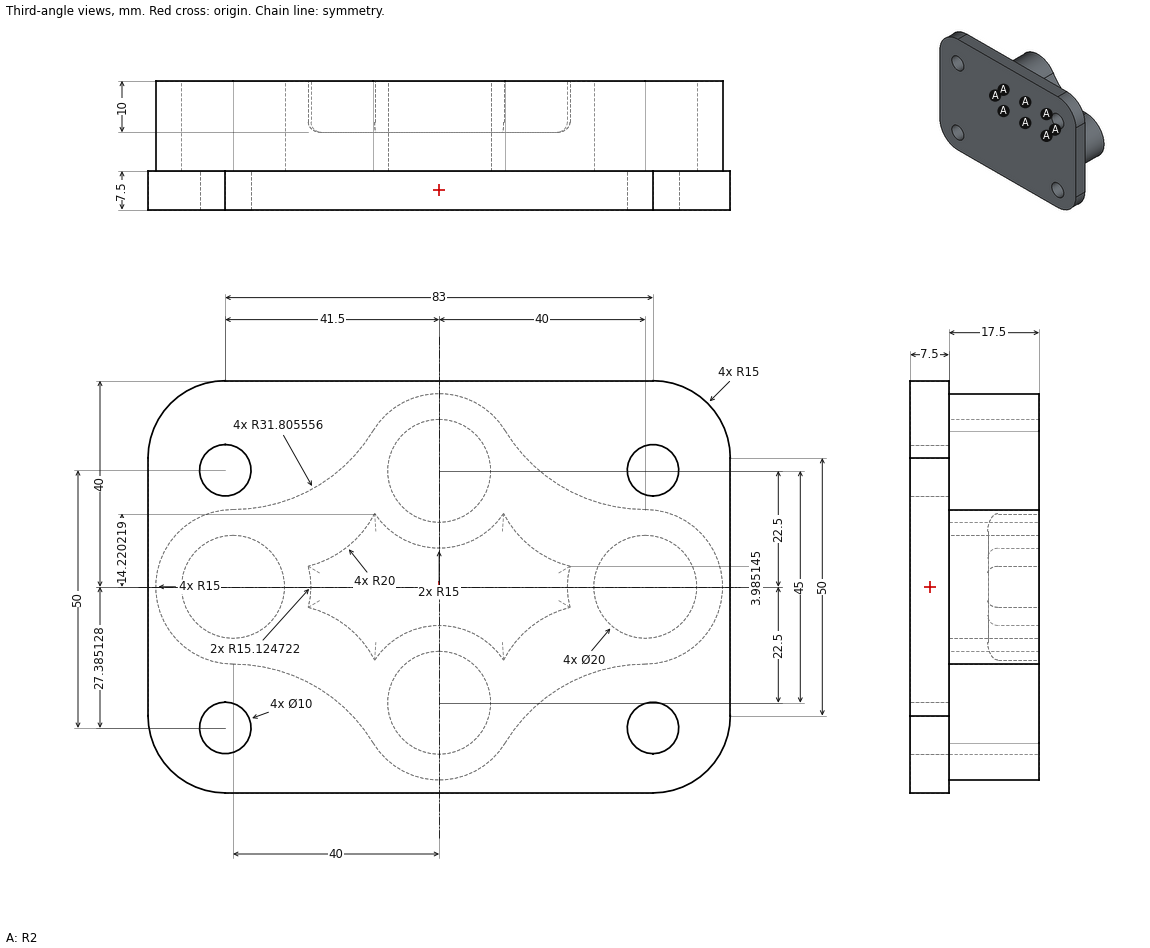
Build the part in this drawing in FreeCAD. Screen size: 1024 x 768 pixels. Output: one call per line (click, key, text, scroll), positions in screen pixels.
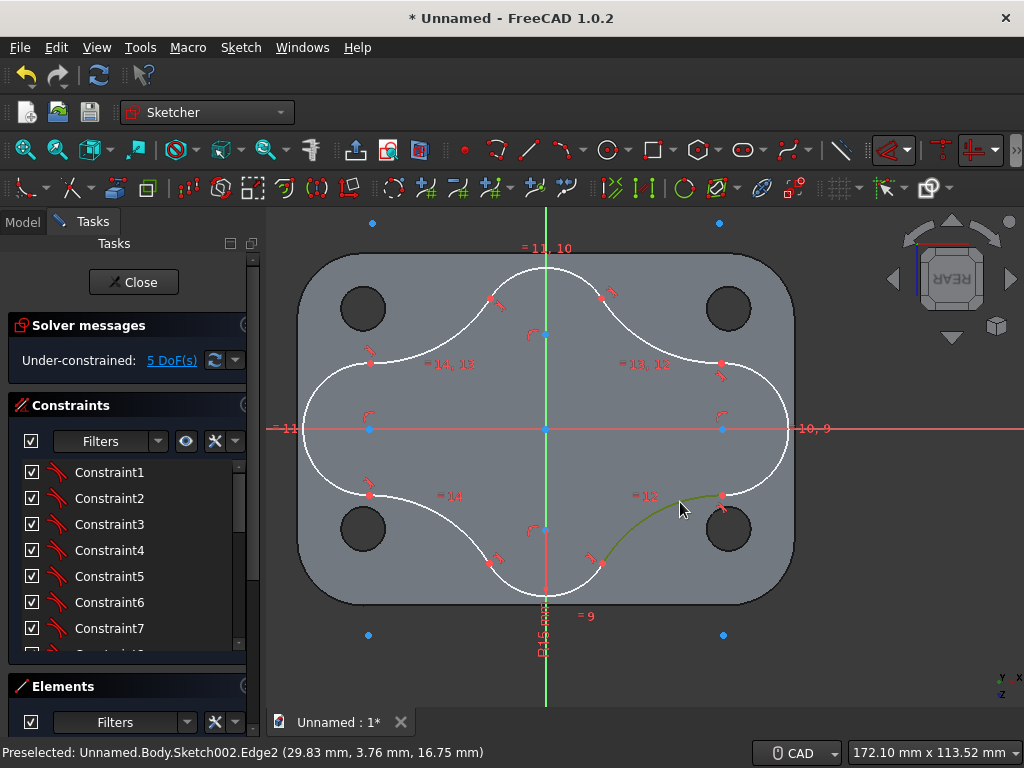
click(910, 150)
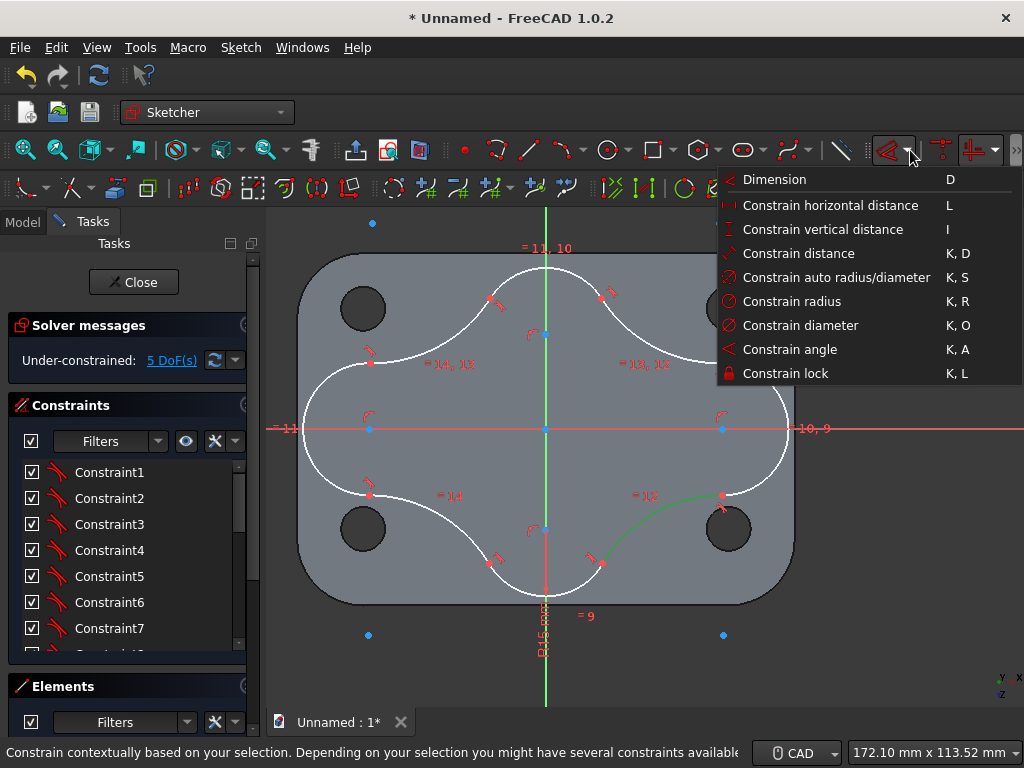
click(870, 301)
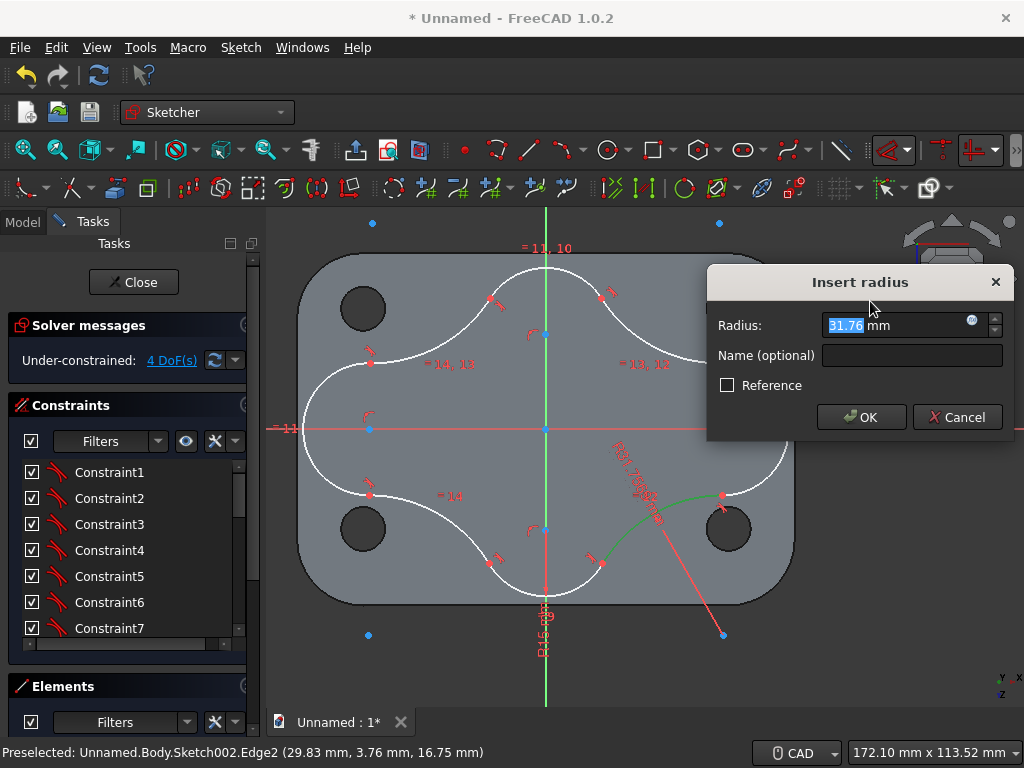
text(31.805556)
key(Return)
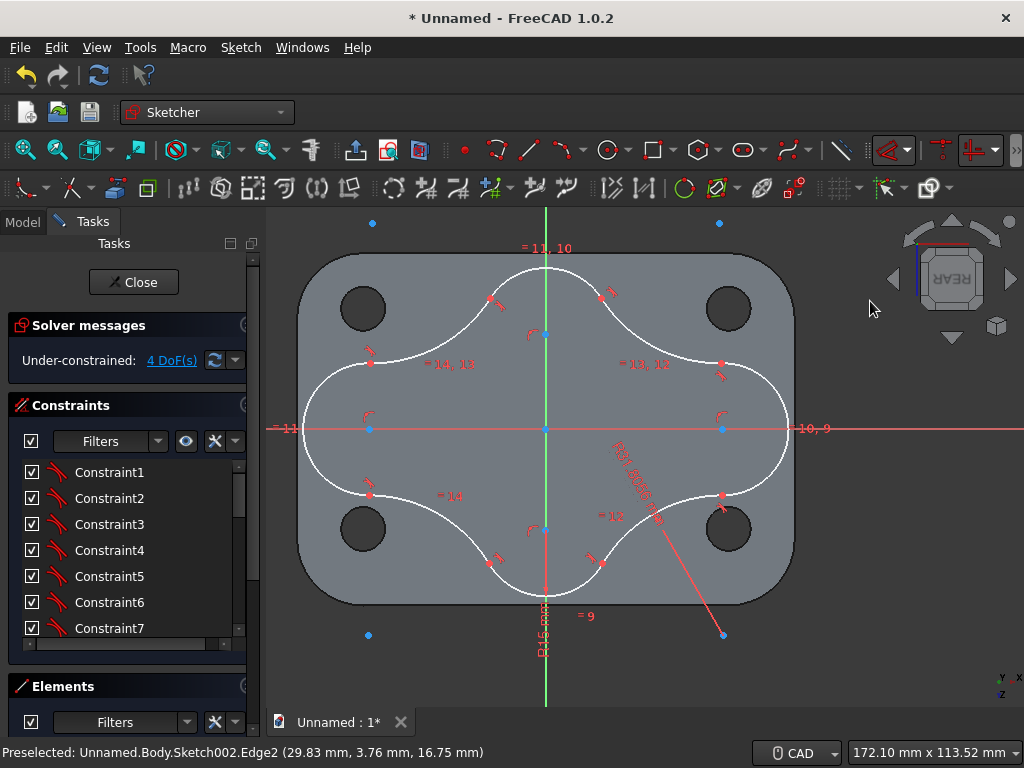
click(723, 495)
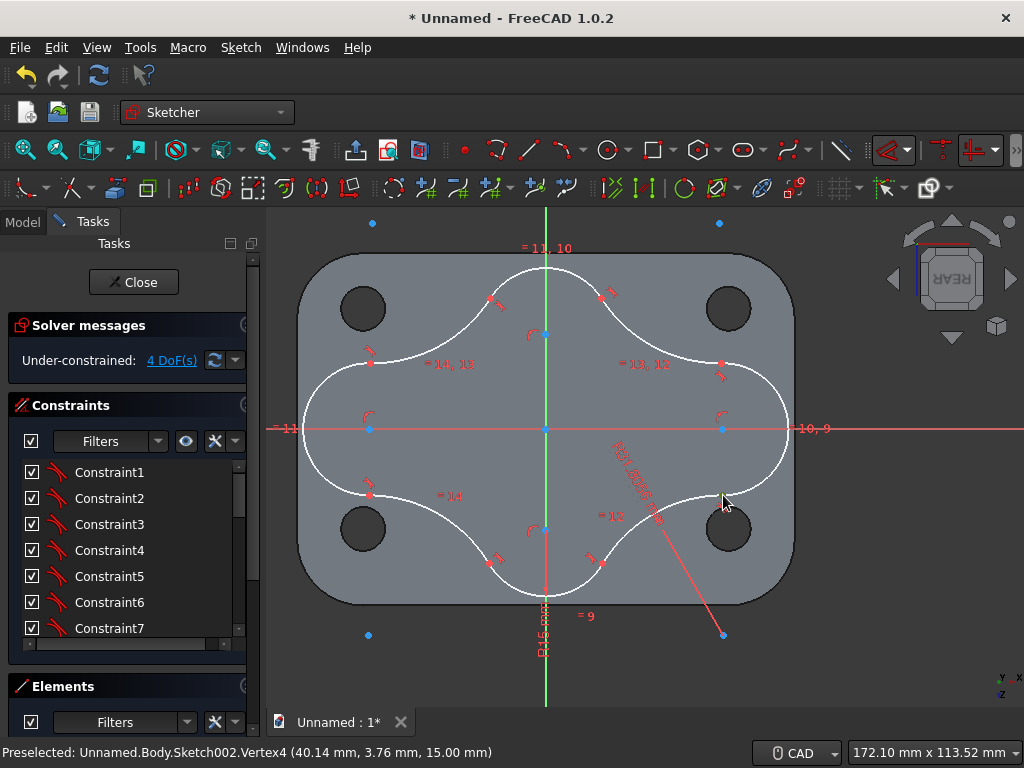
click(910, 150)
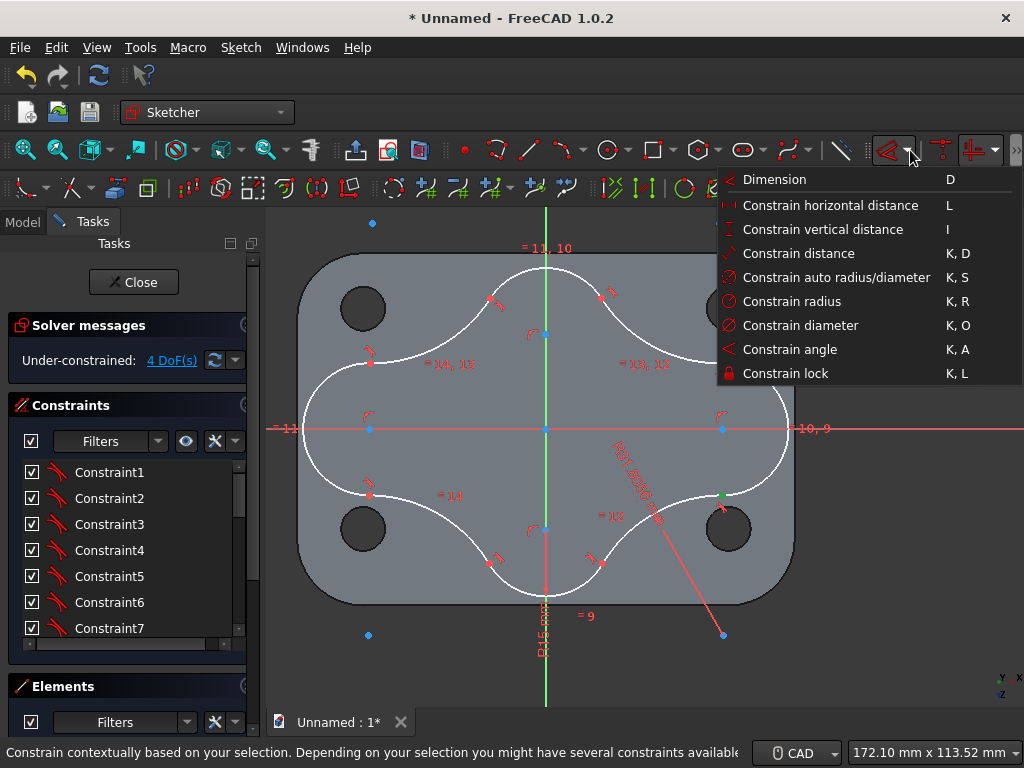
click(870, 205)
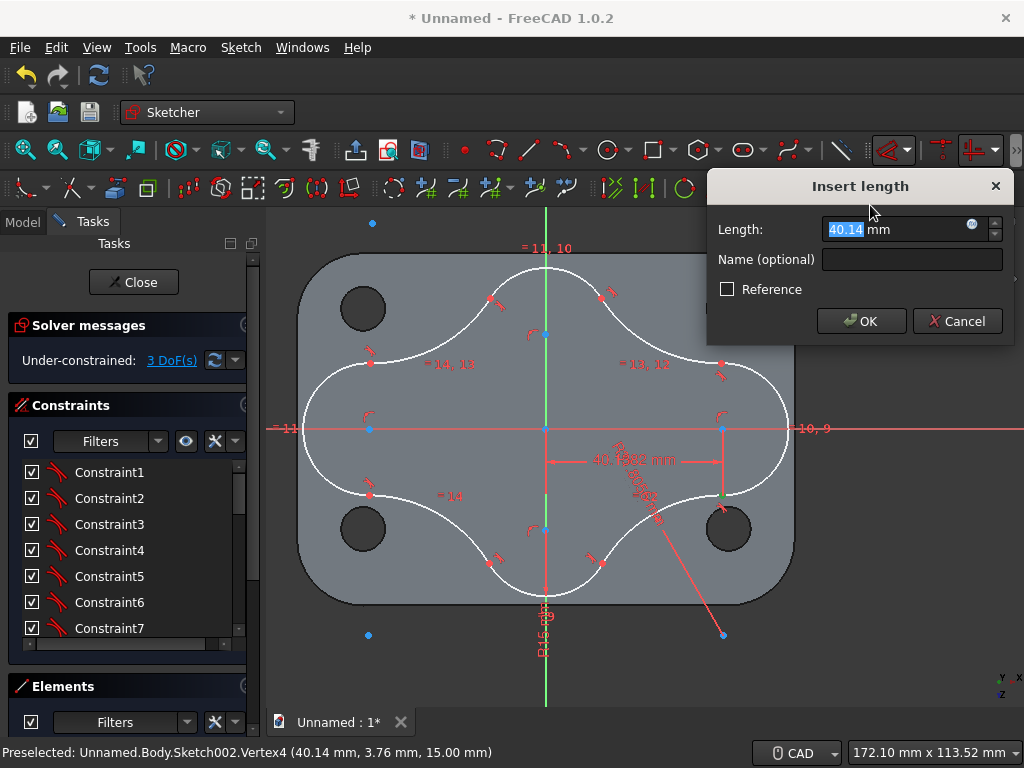
text(40)
key(Return)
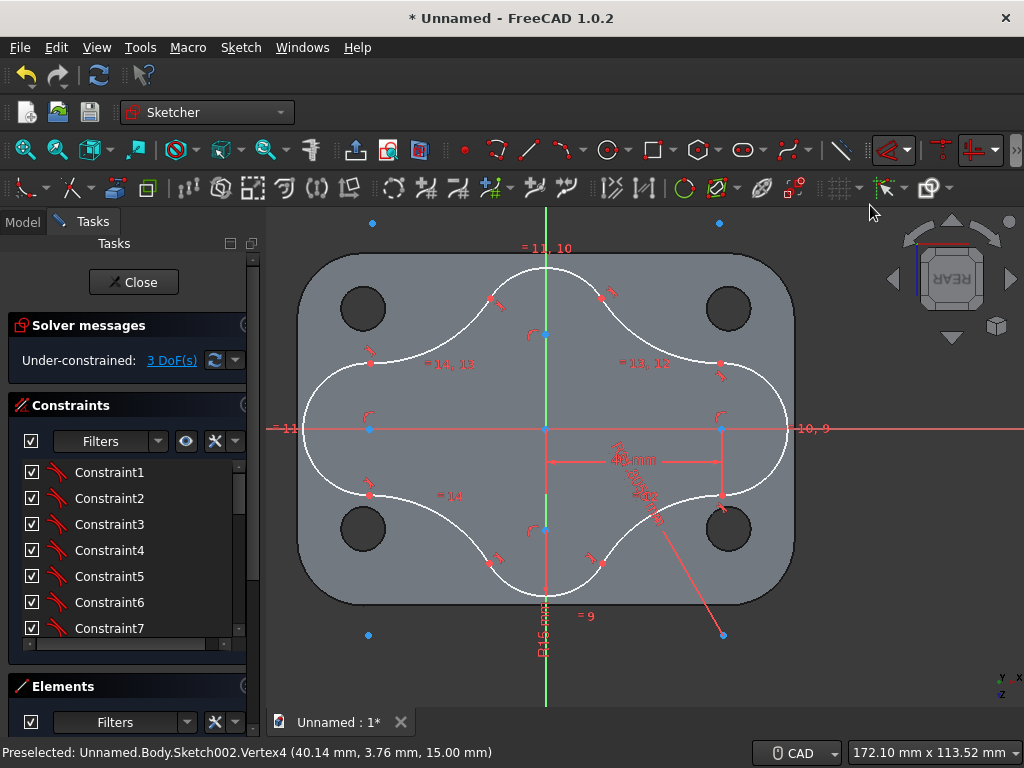
click(370, 363)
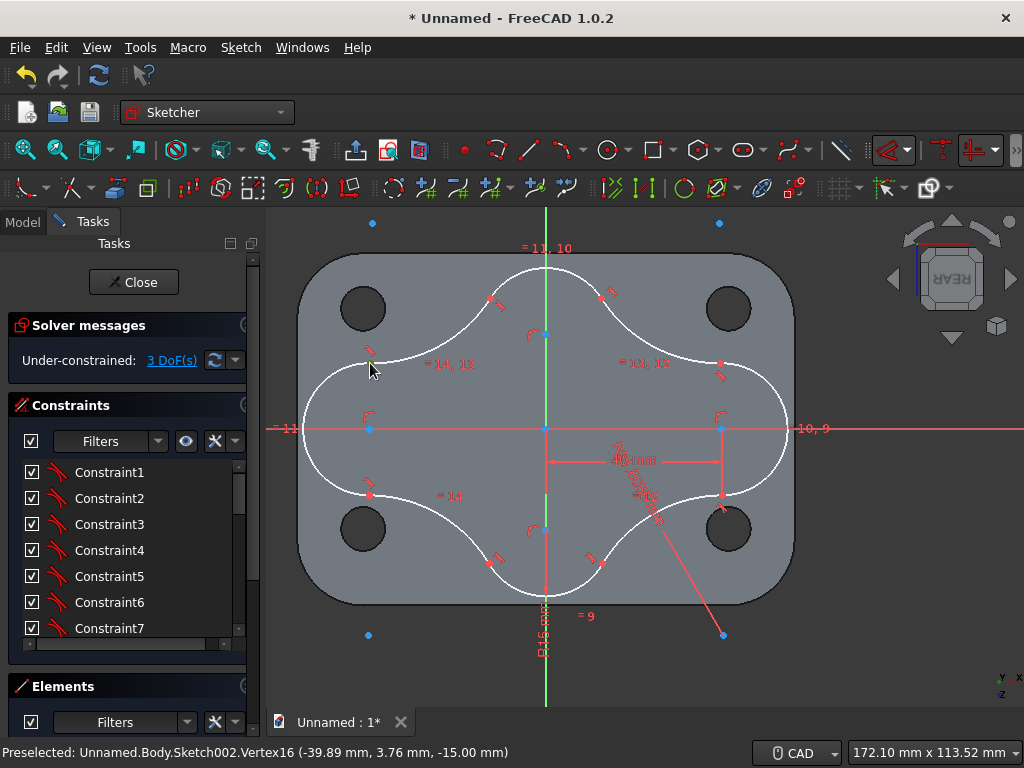
click(910, 150)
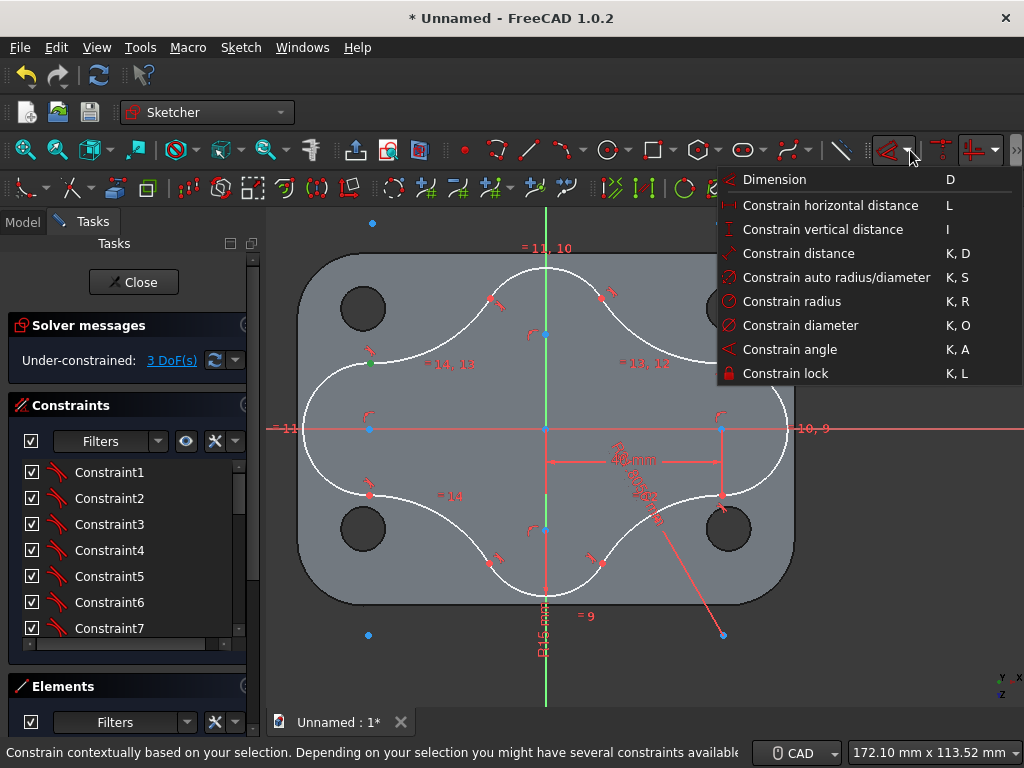
click(870, 205)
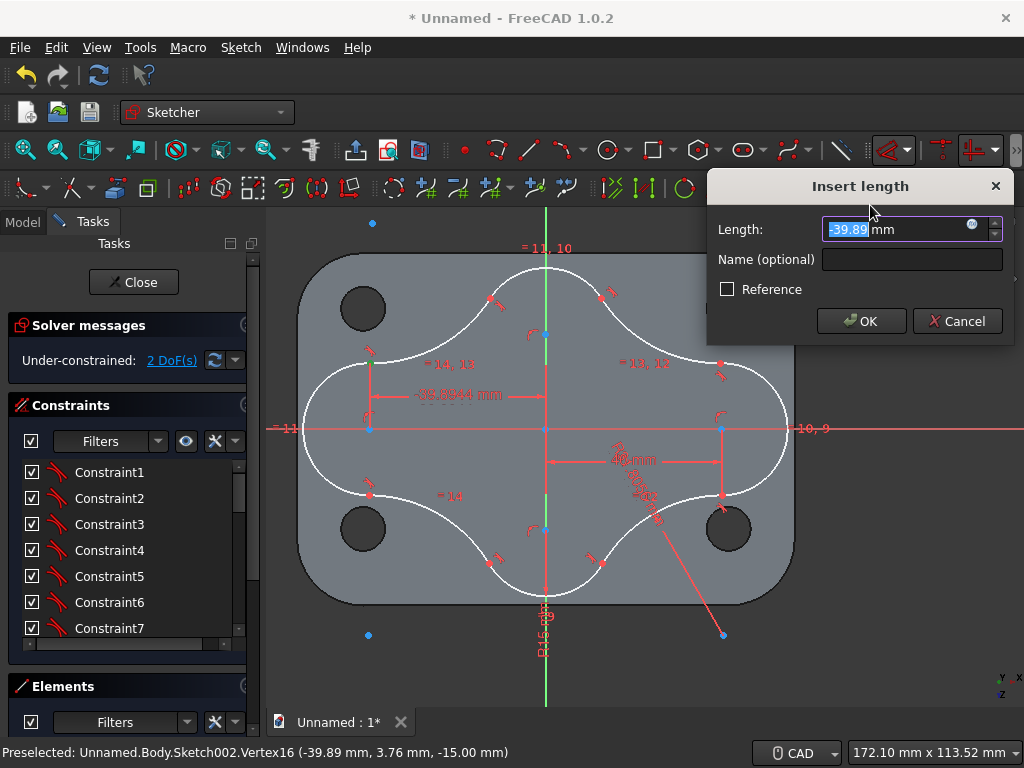
text(-40)
key(Return)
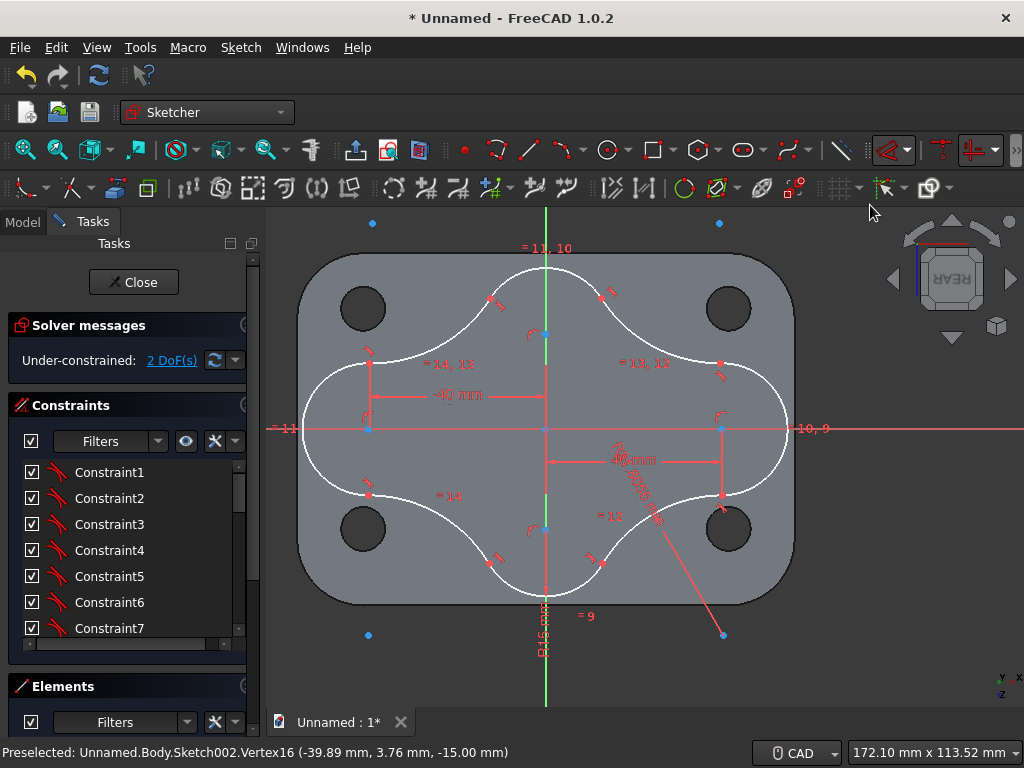
click(723, 635)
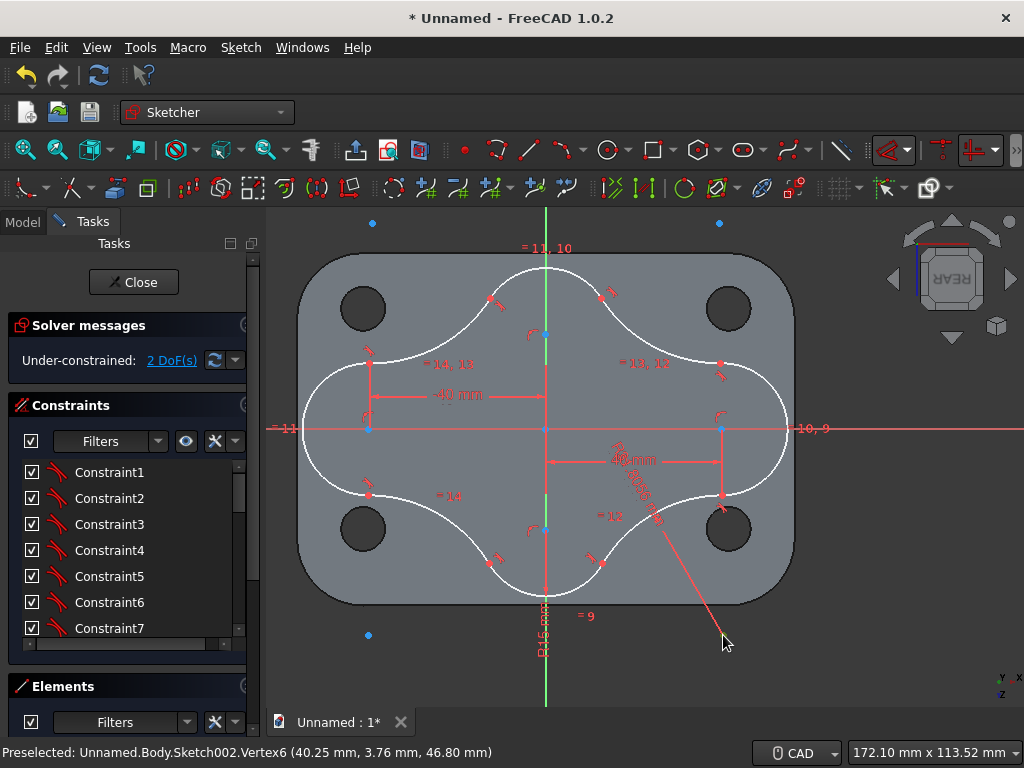
click(910, 150)